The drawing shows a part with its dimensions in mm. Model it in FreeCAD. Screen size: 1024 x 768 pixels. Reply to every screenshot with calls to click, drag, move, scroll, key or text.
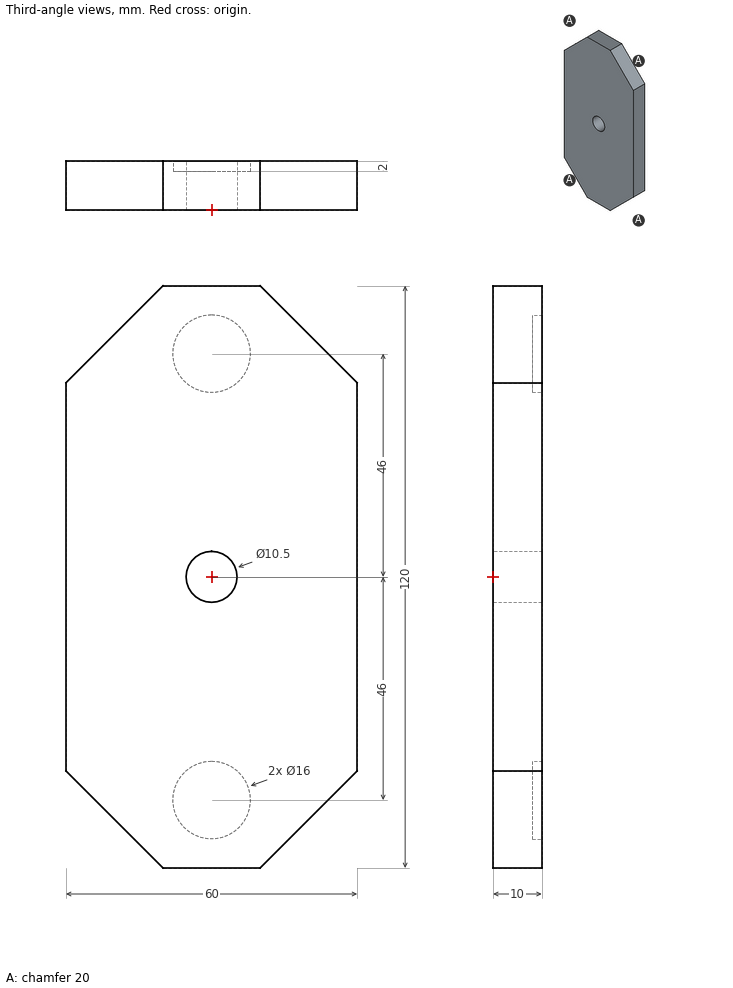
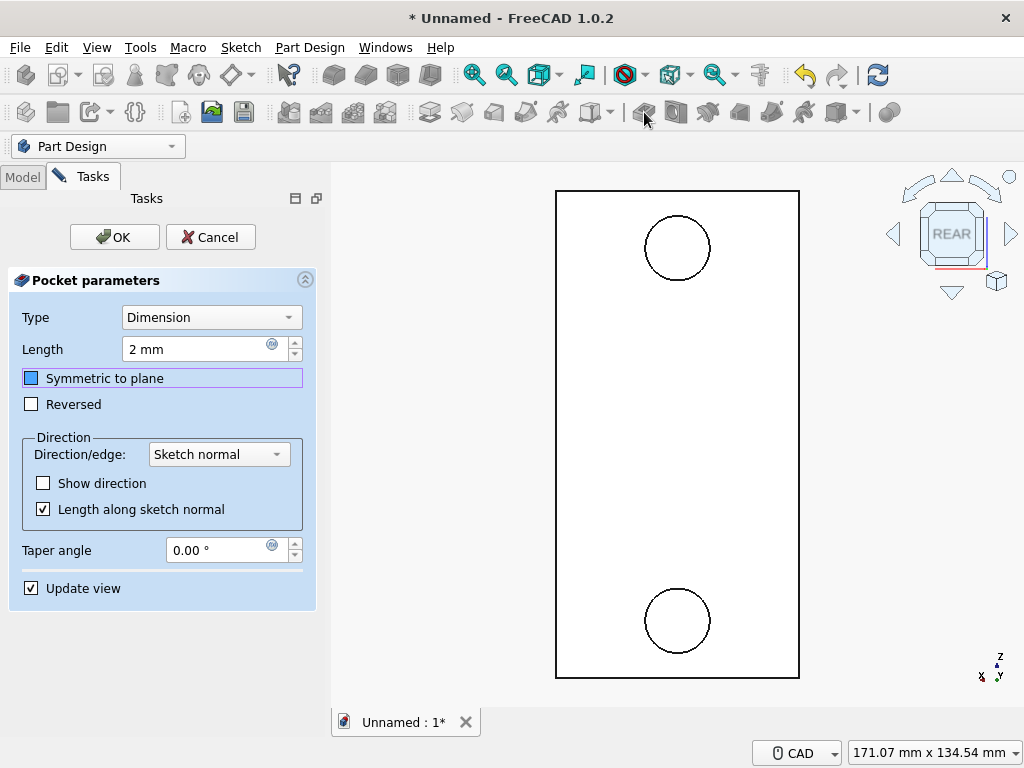
click(115, 237)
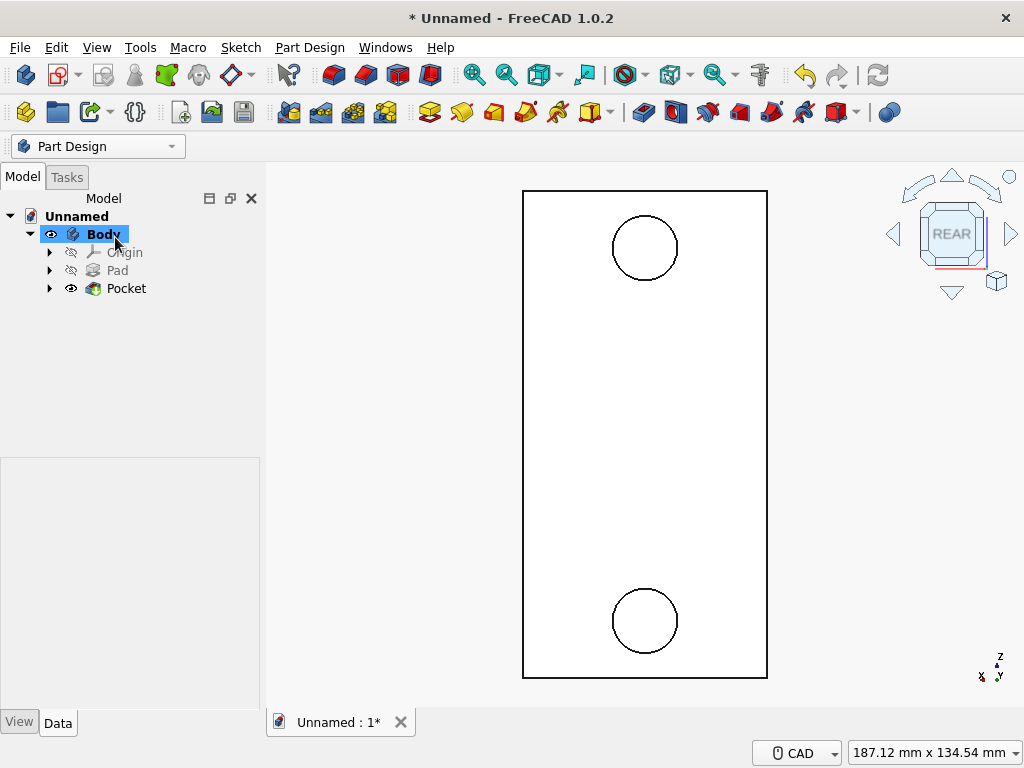
key(0)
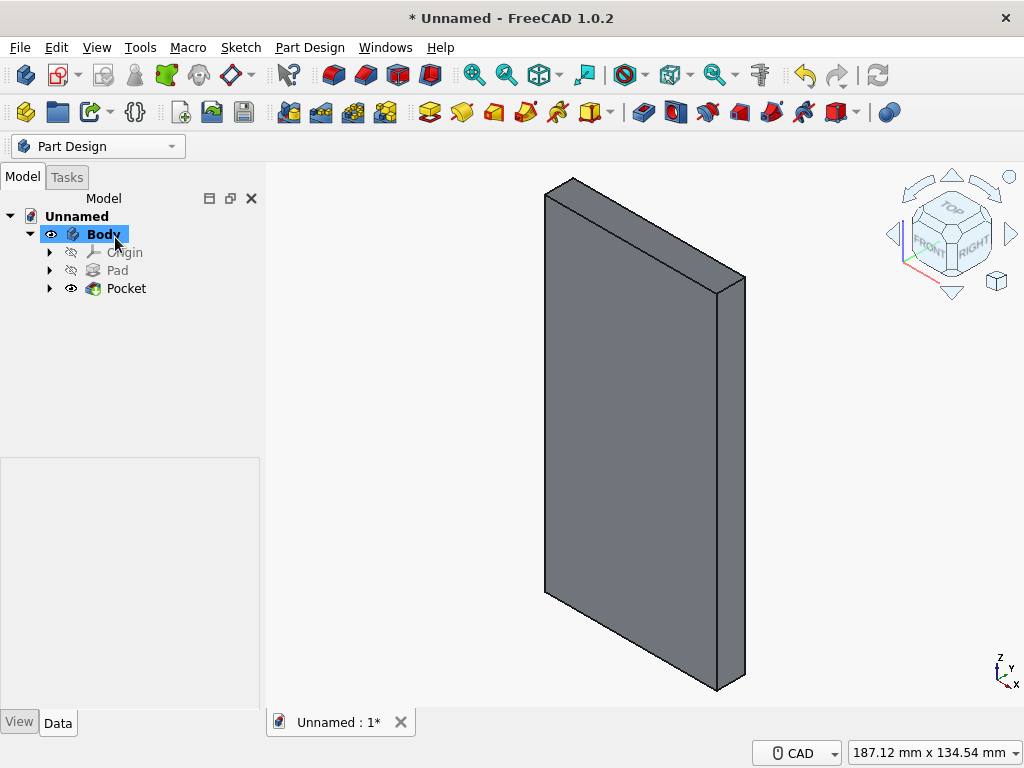
click(731, 285)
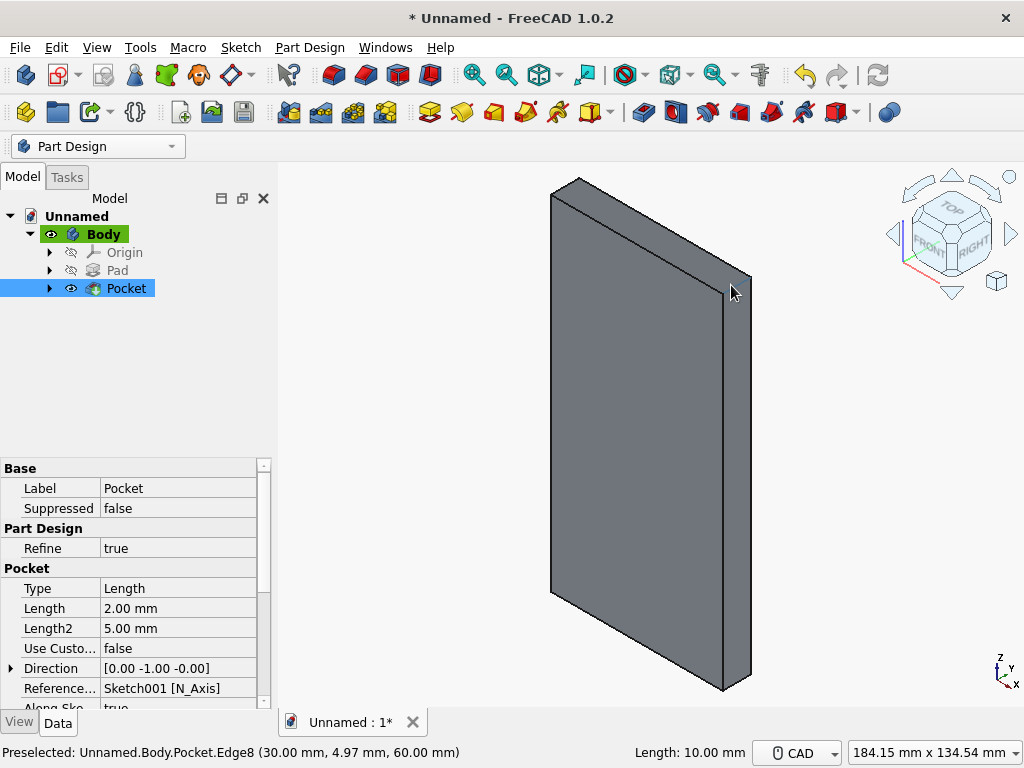
key(2)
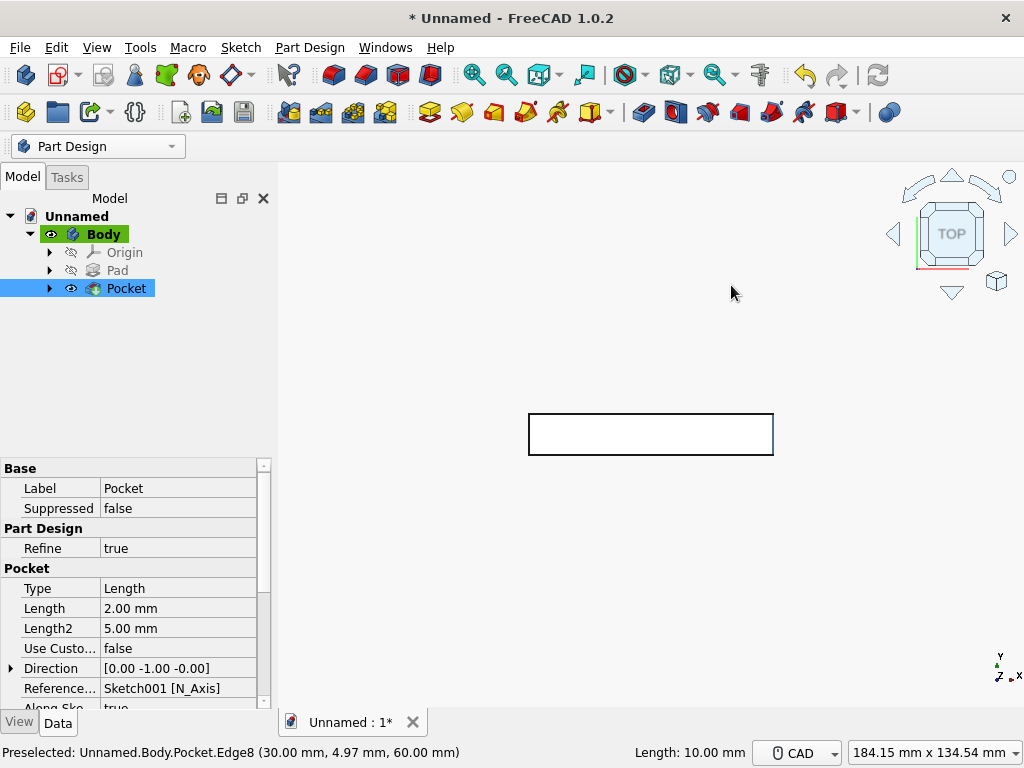
click(476, 76)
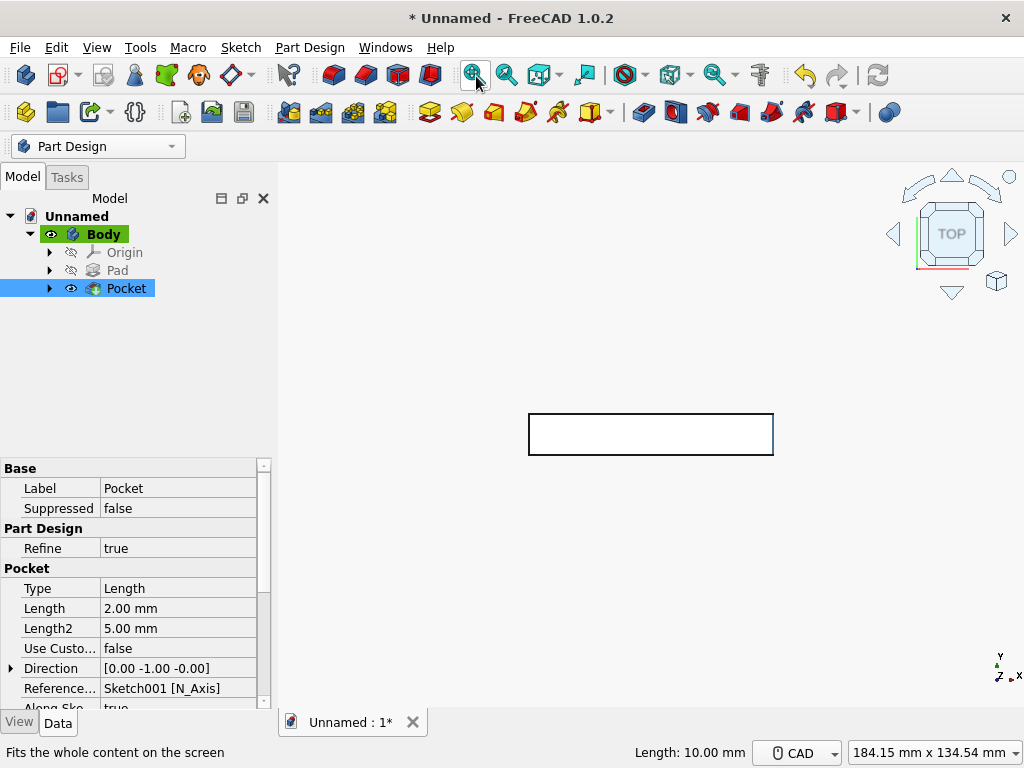
click(529, 433, ctrl)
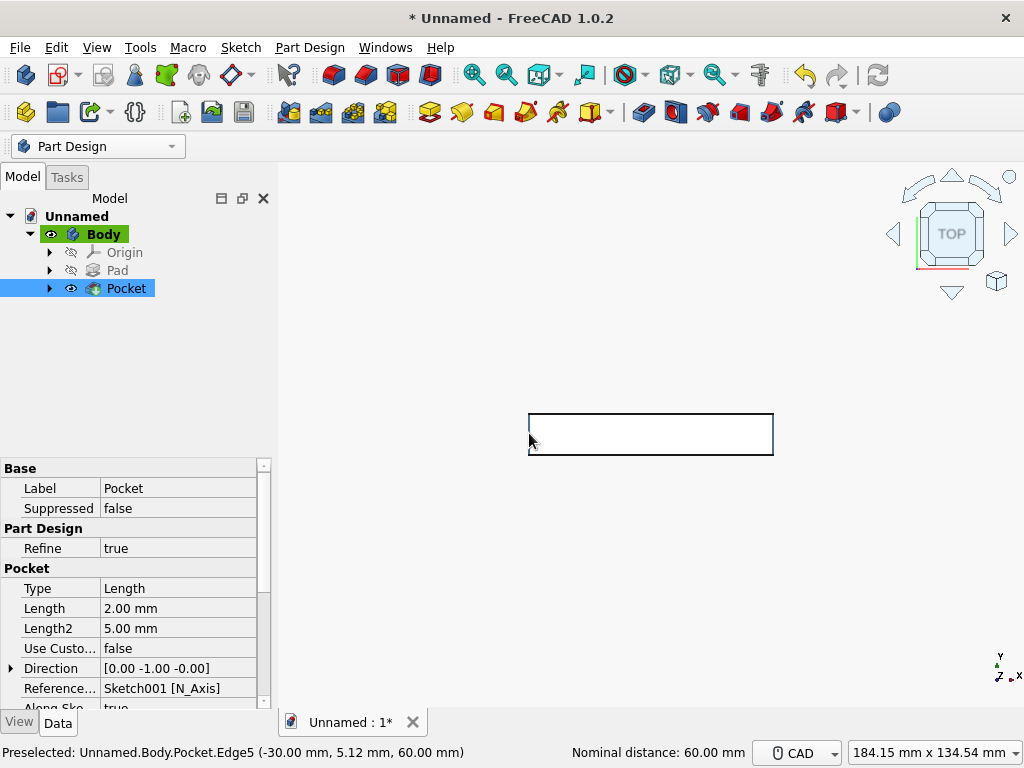
key(1)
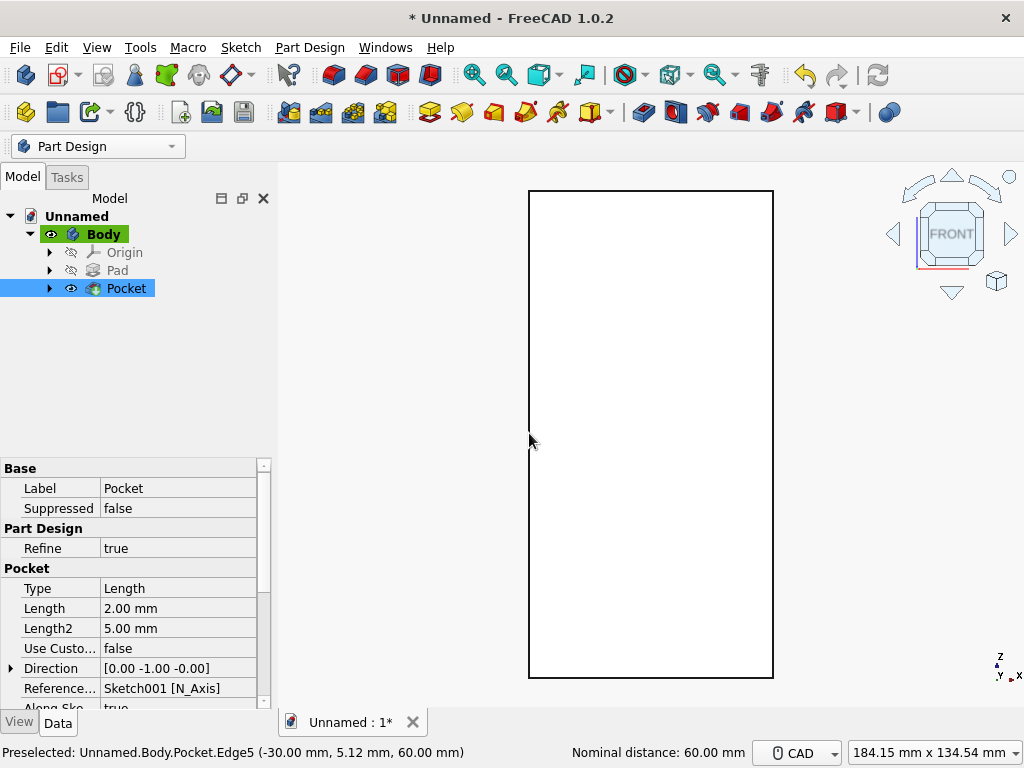
key(3)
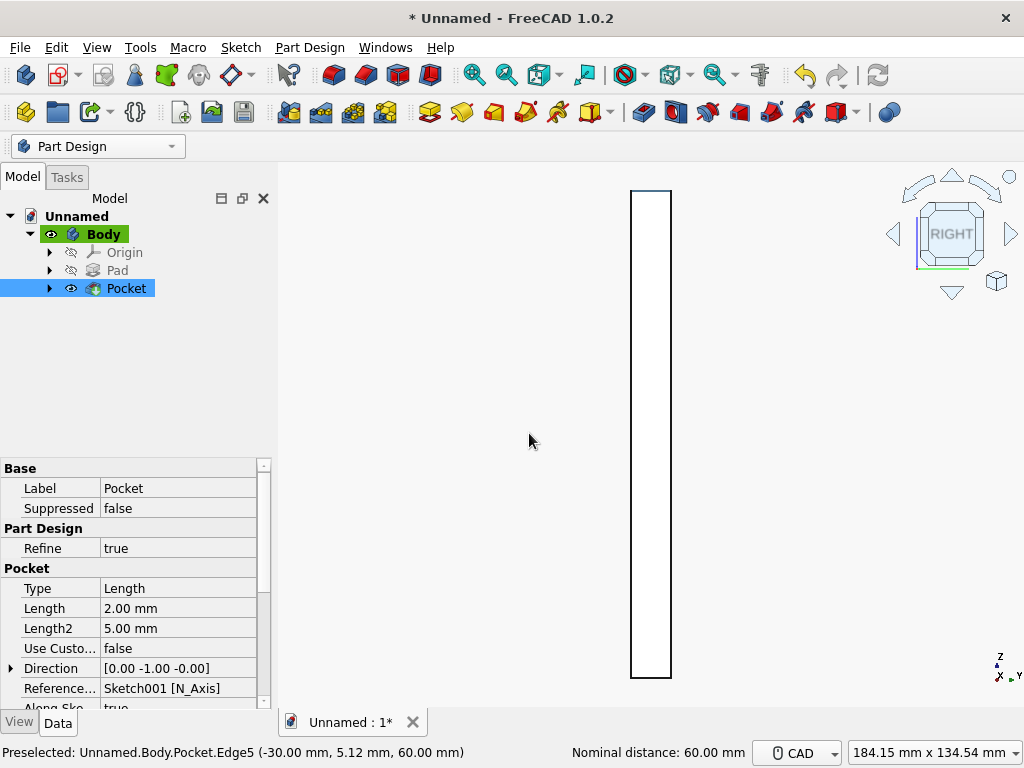
click(651, 677, ctrl)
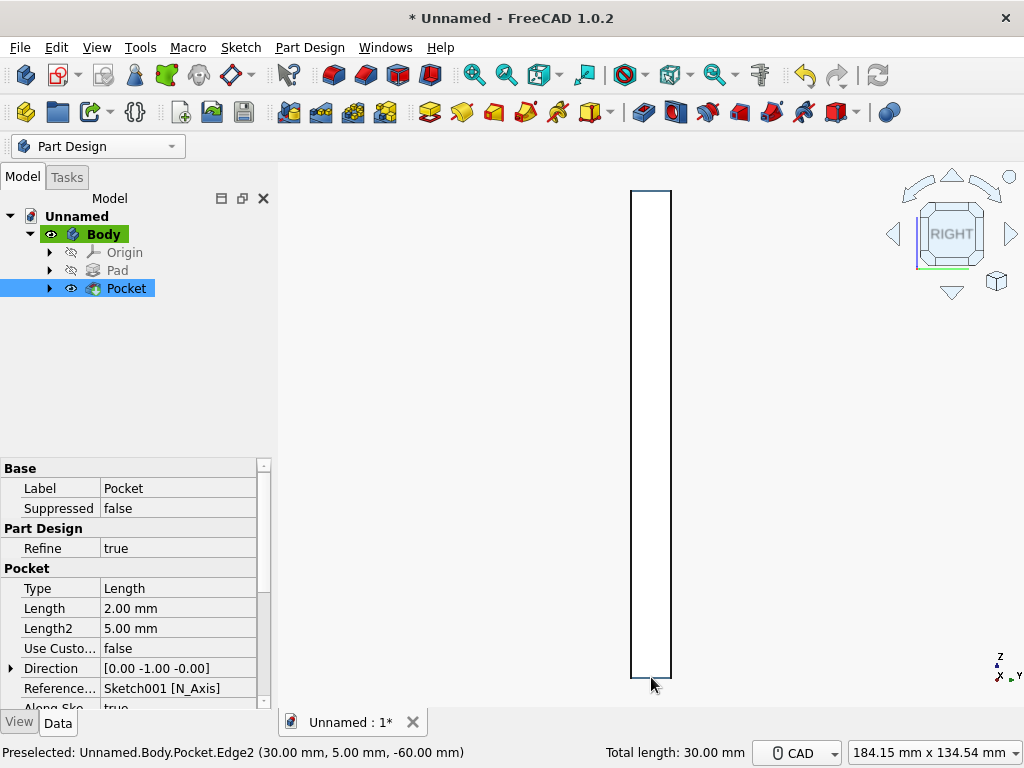
key(5)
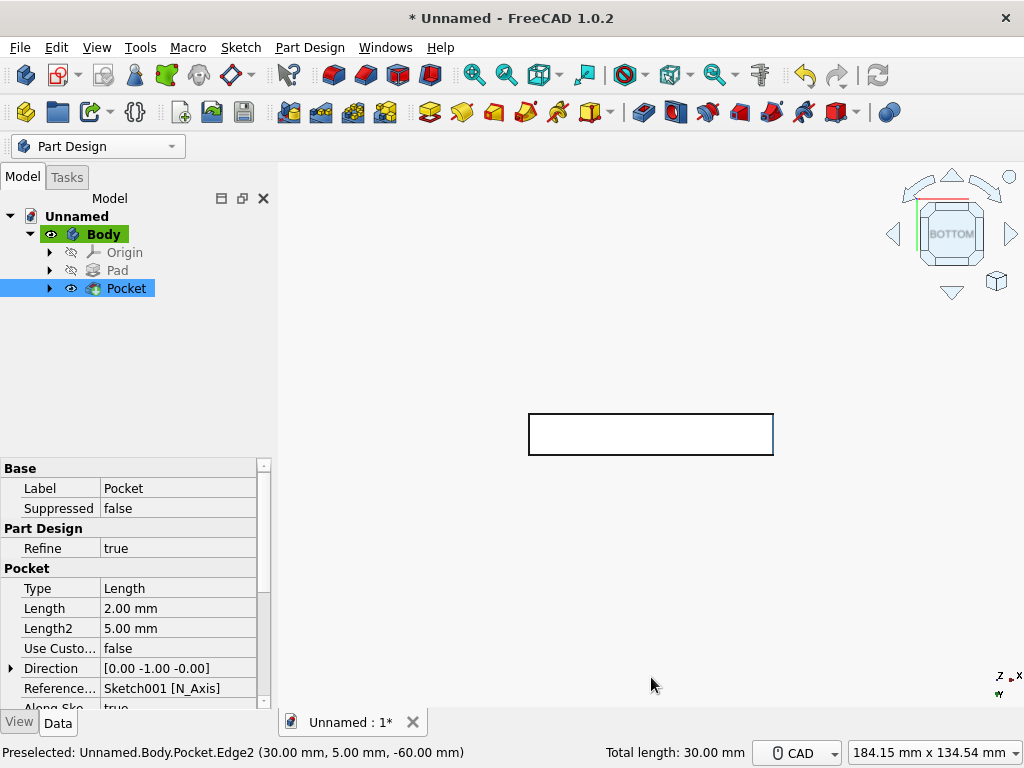
click(476, 76)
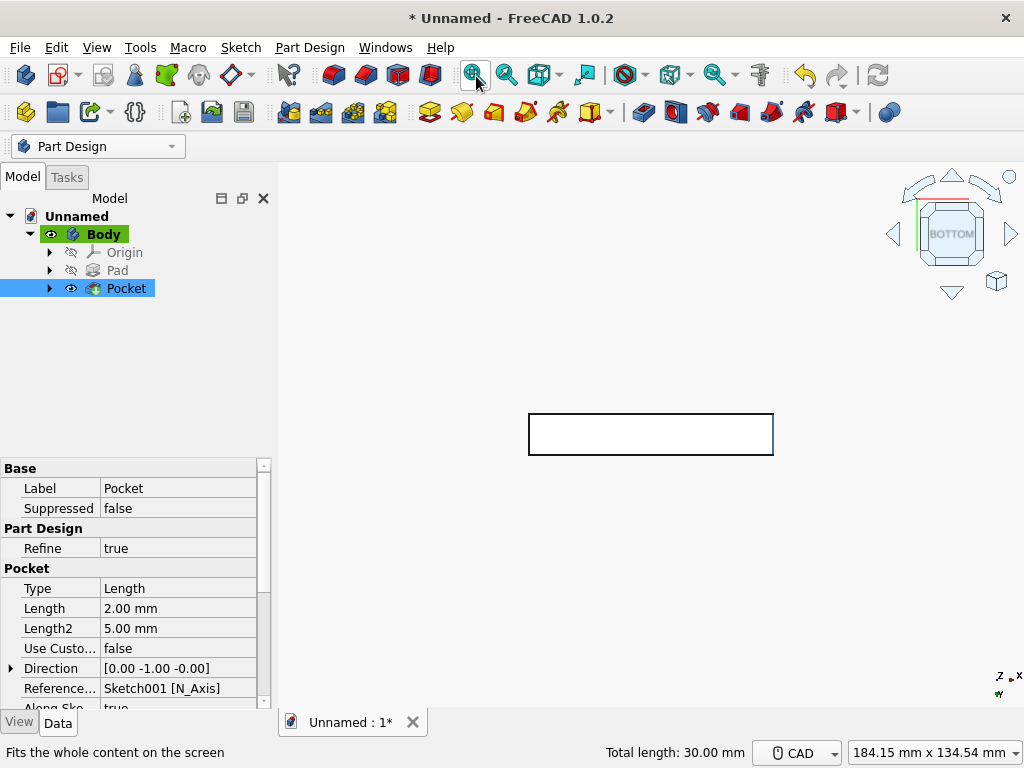
click(529, 433, ctrl)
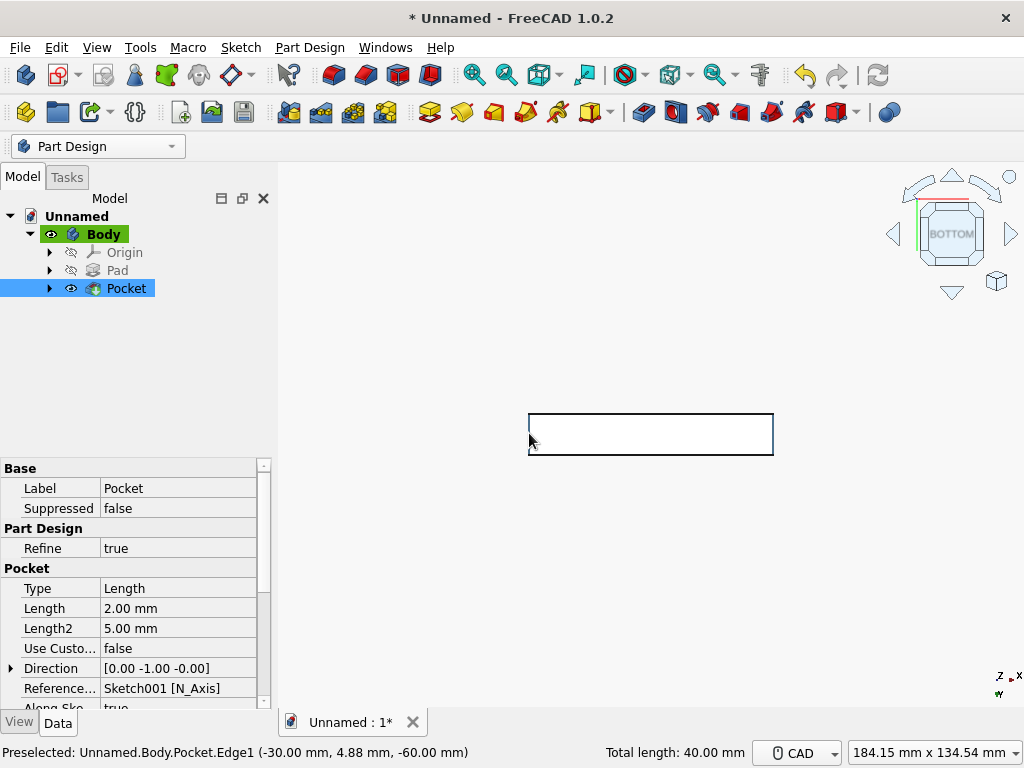
click(366, 76)